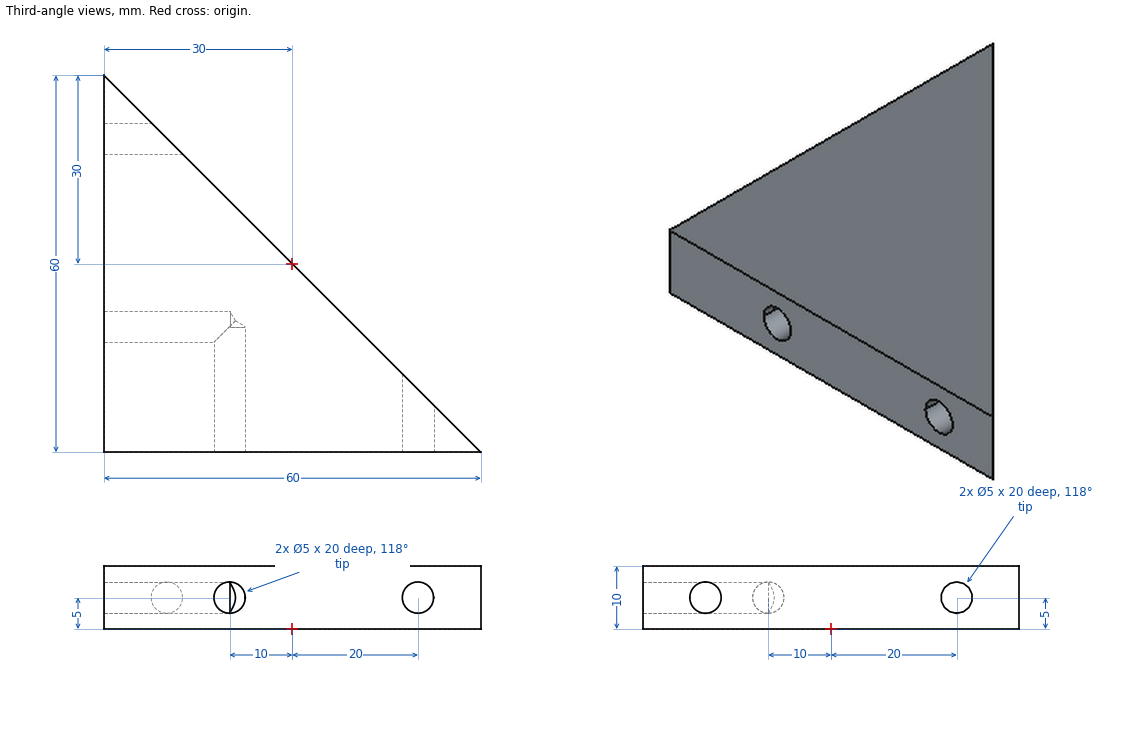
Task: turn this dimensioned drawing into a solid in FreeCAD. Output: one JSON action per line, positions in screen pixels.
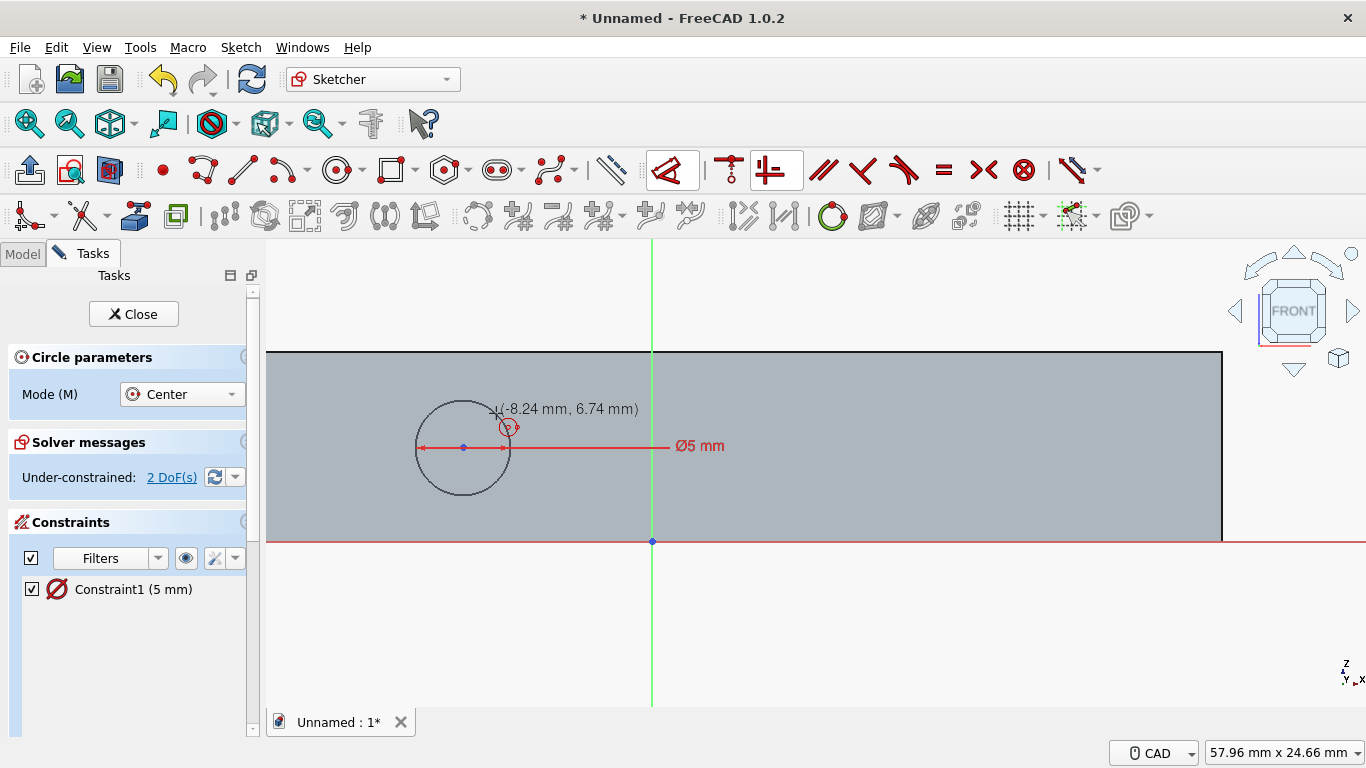
{"action": "left_click", "coordinate": [1032, 447]}
{"action": "mouse_move", "coordinate": [1066, 413]}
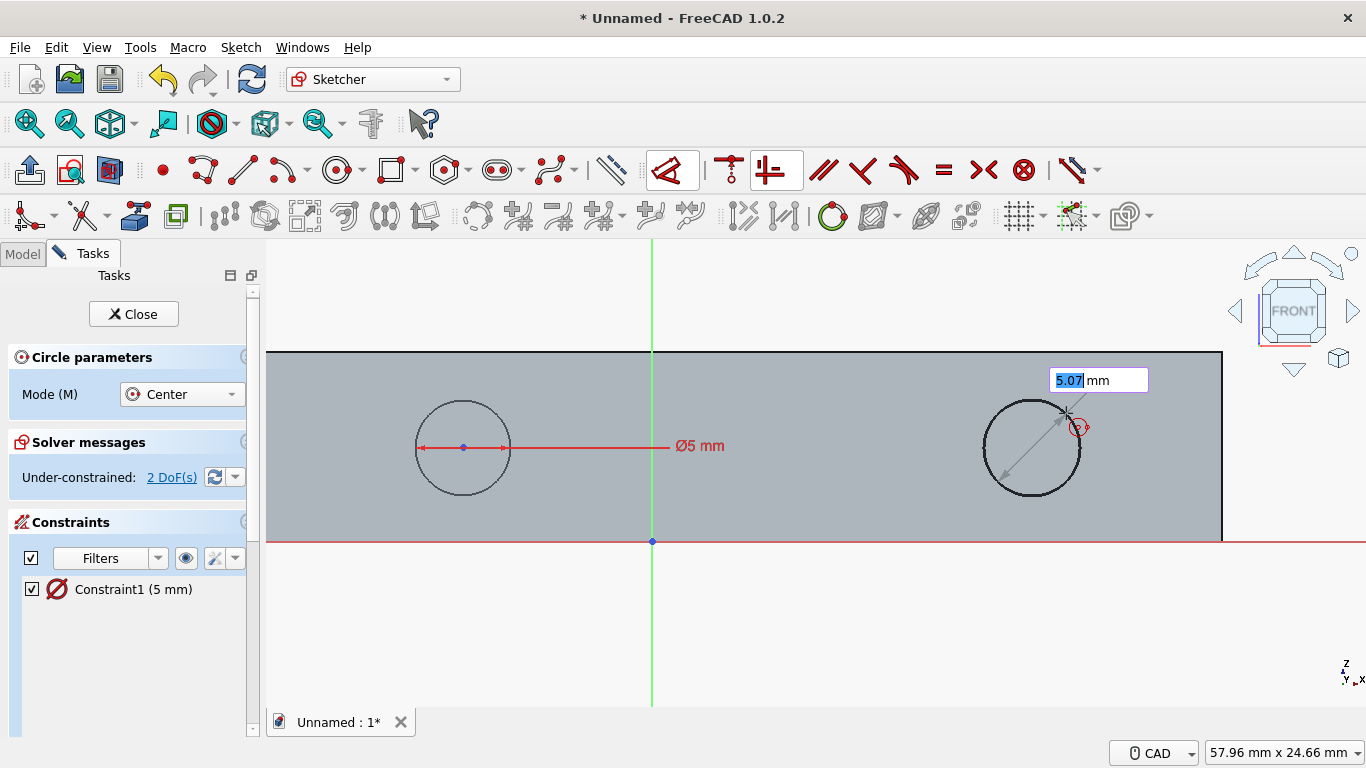
{"action": "type", "text": "5"}
{"action": "key", "text": "Return"}
{"action": "key", "text": "Escape"}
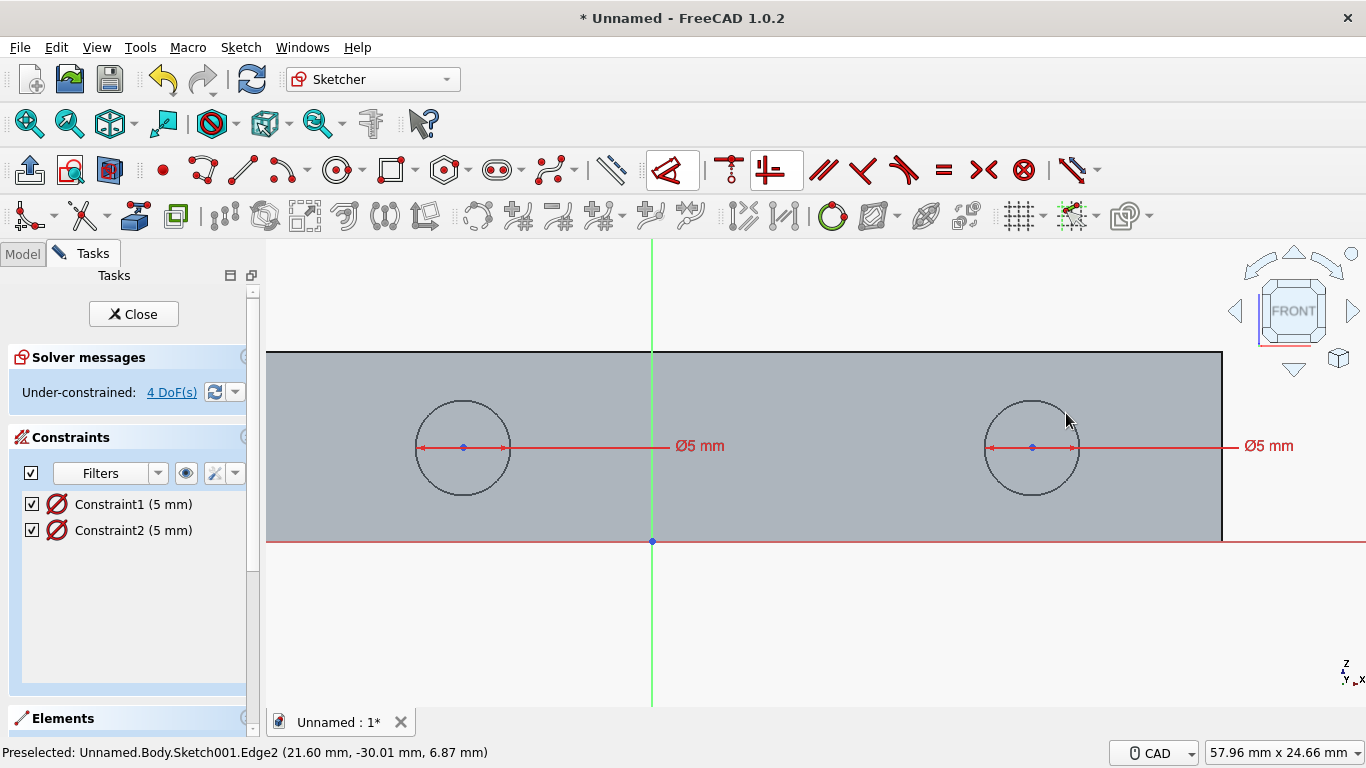
{"action": "left_click", "coordinate": [463, 448]}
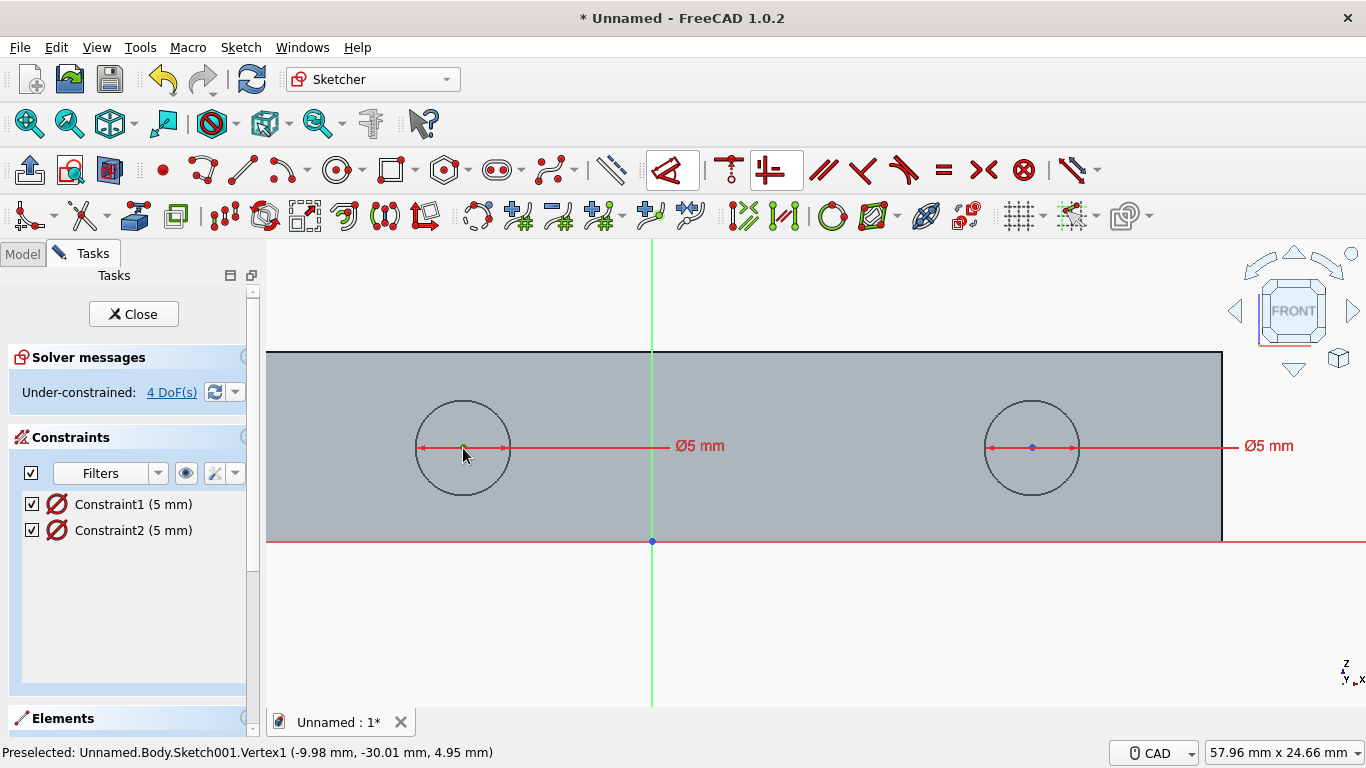
{"action": "left_click", "coordinate": [694, 170]}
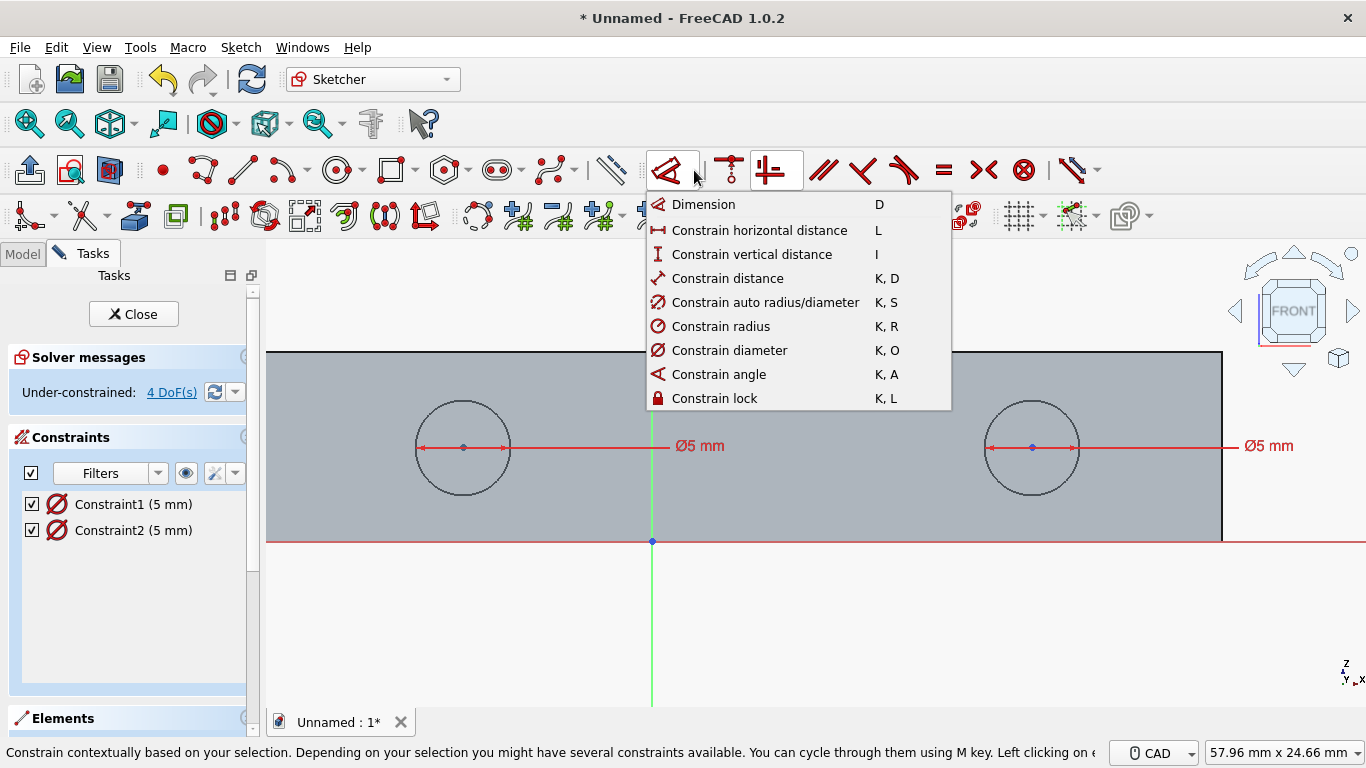
{"action": "left_click", "coordinate": [799, 254]}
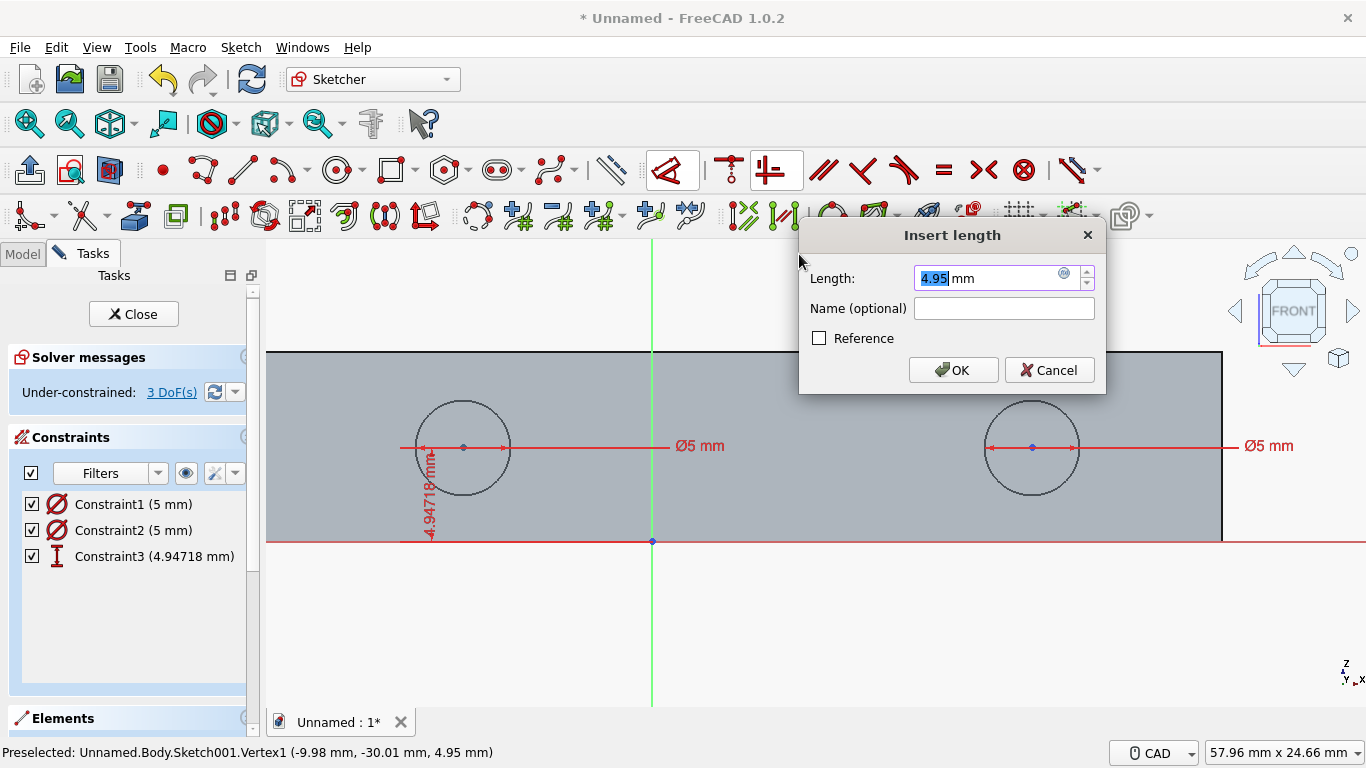
{"action": "type", "text": "5"}
{"action": "key", "text": "Return"}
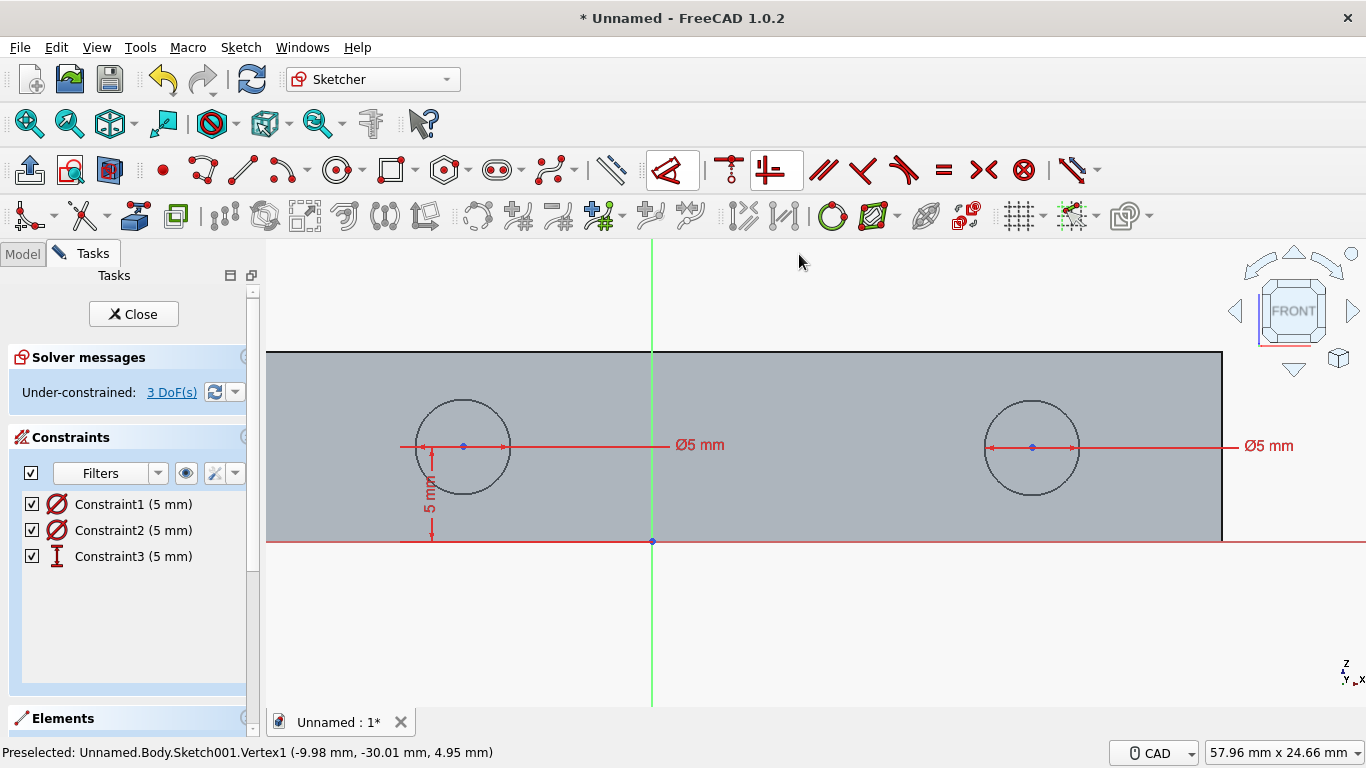
{"action": "left_click", "coordinate": [1032, 448]}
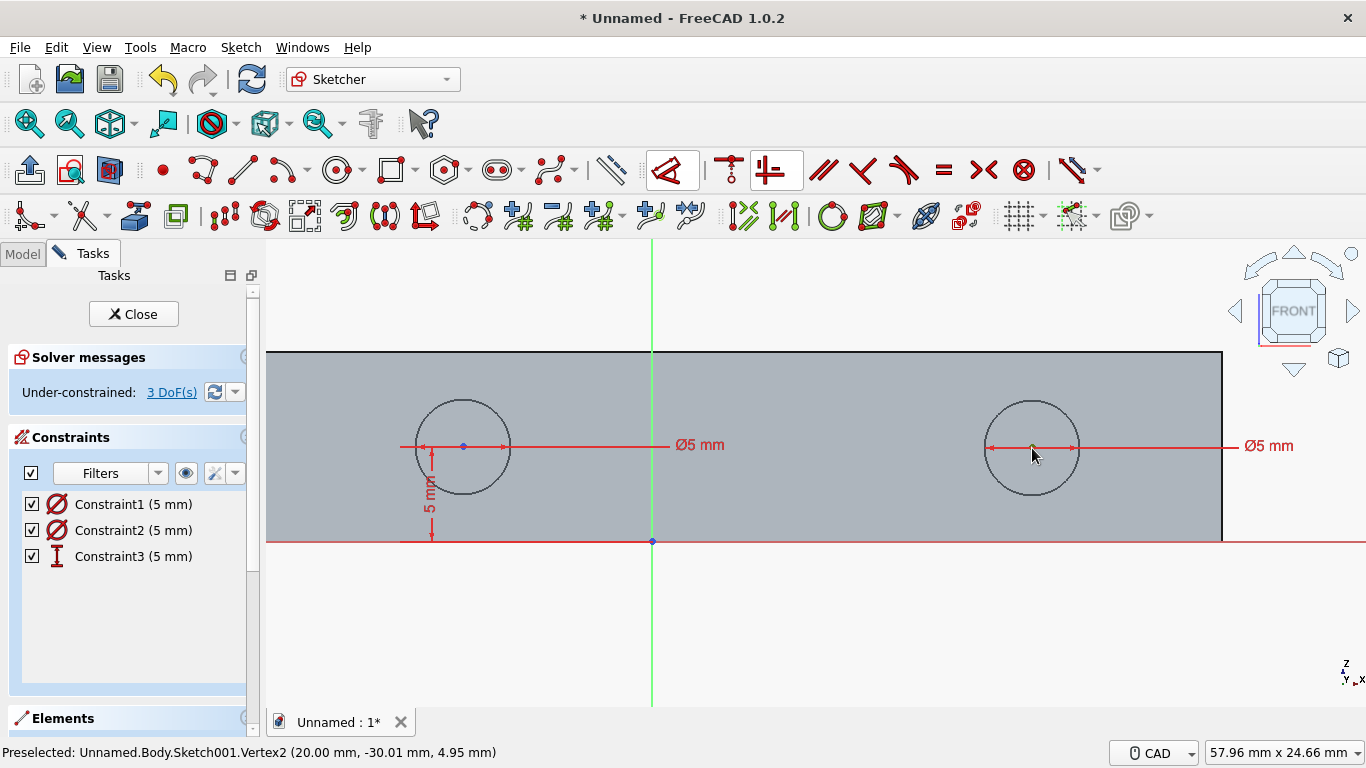
{"action": "key", "text": "i"}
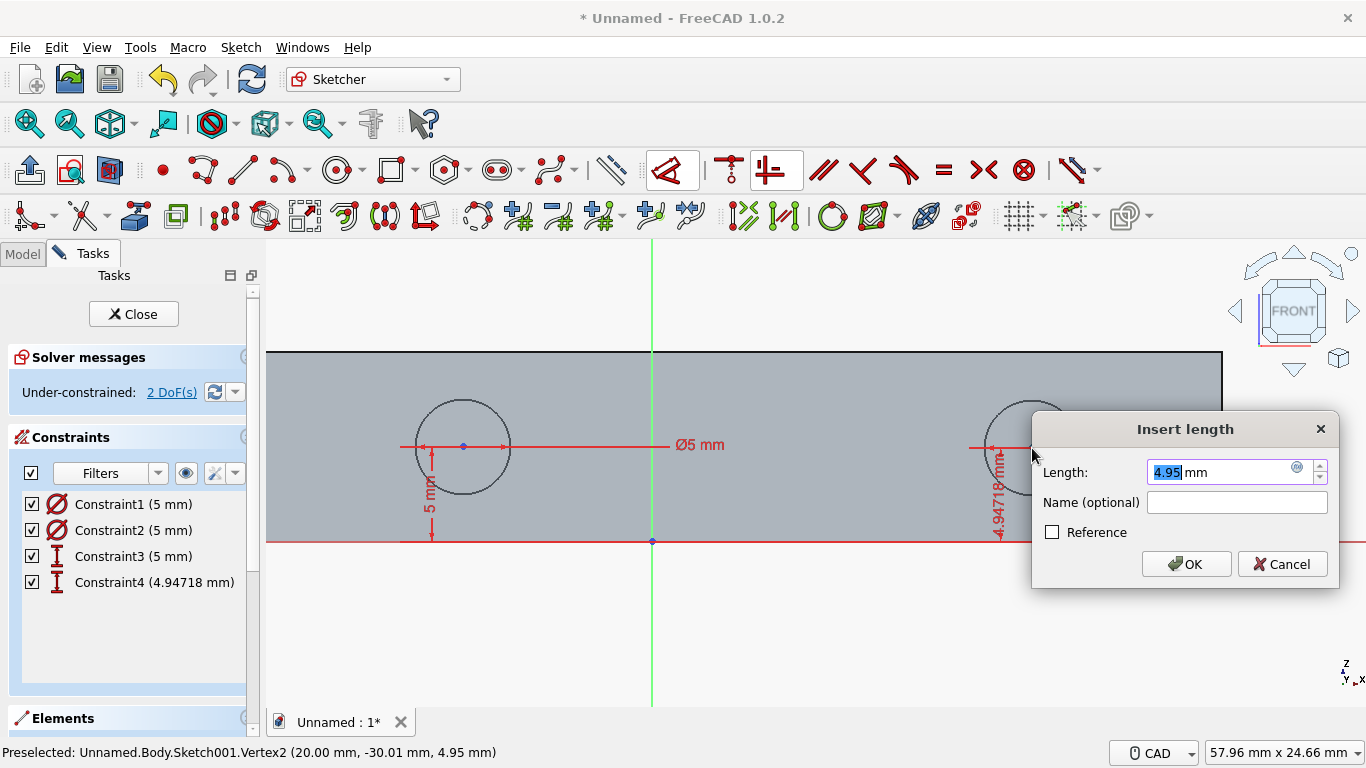
{"action": "type", "text": "5"}
{"action": "key", "text": "Return"}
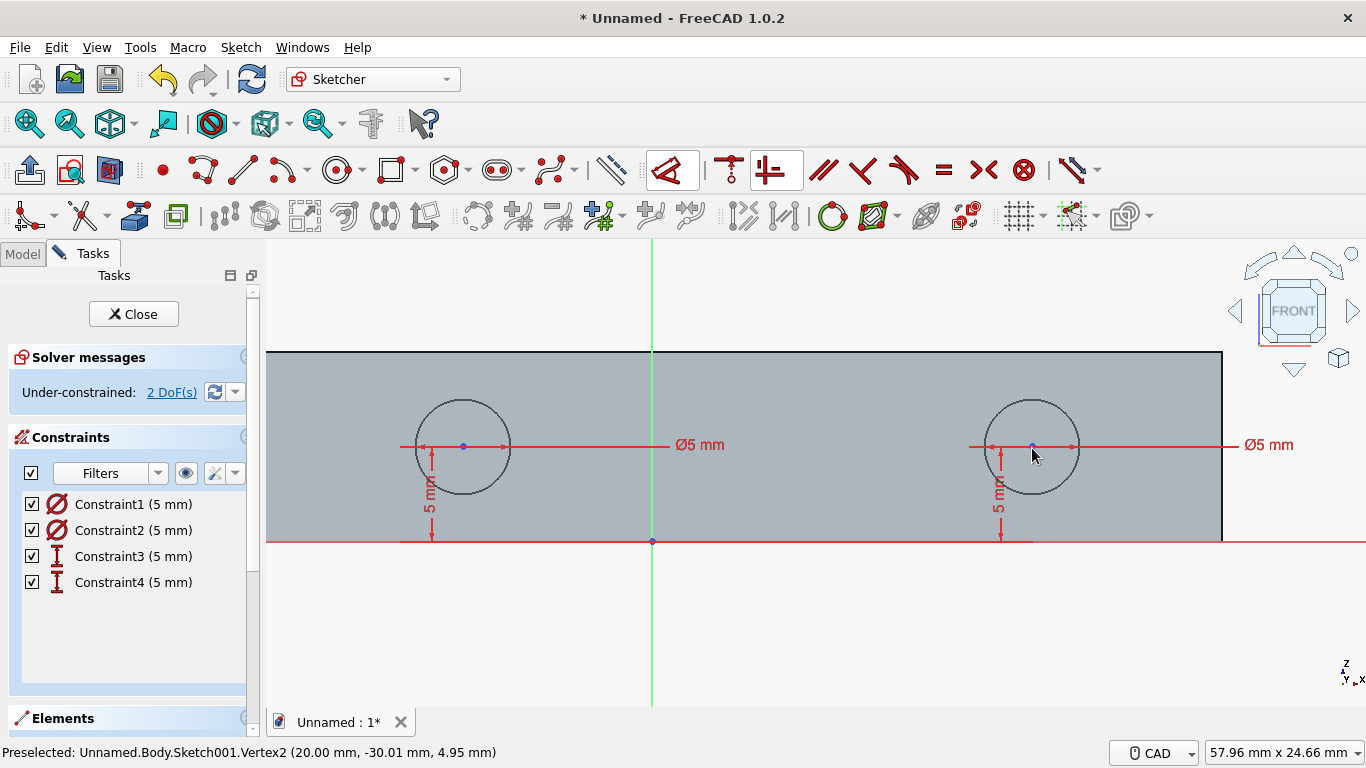
{"action": "left_click", "coordinate": [463, 447]}